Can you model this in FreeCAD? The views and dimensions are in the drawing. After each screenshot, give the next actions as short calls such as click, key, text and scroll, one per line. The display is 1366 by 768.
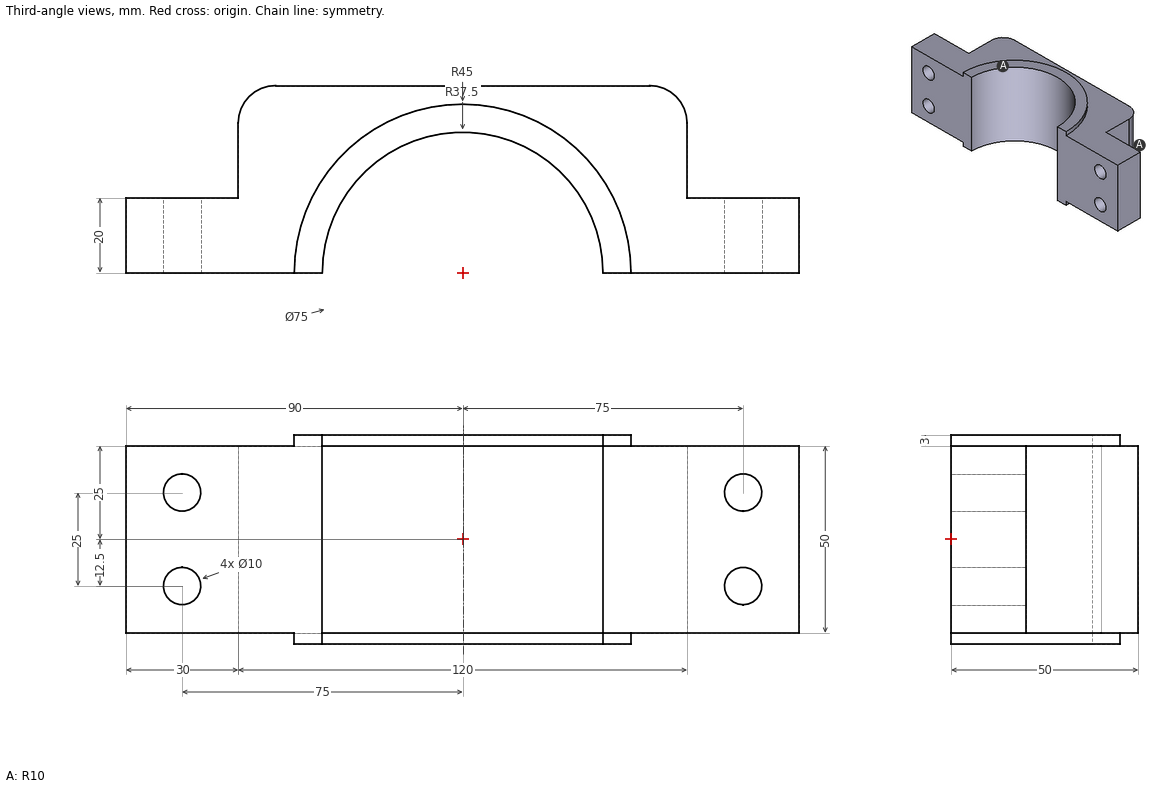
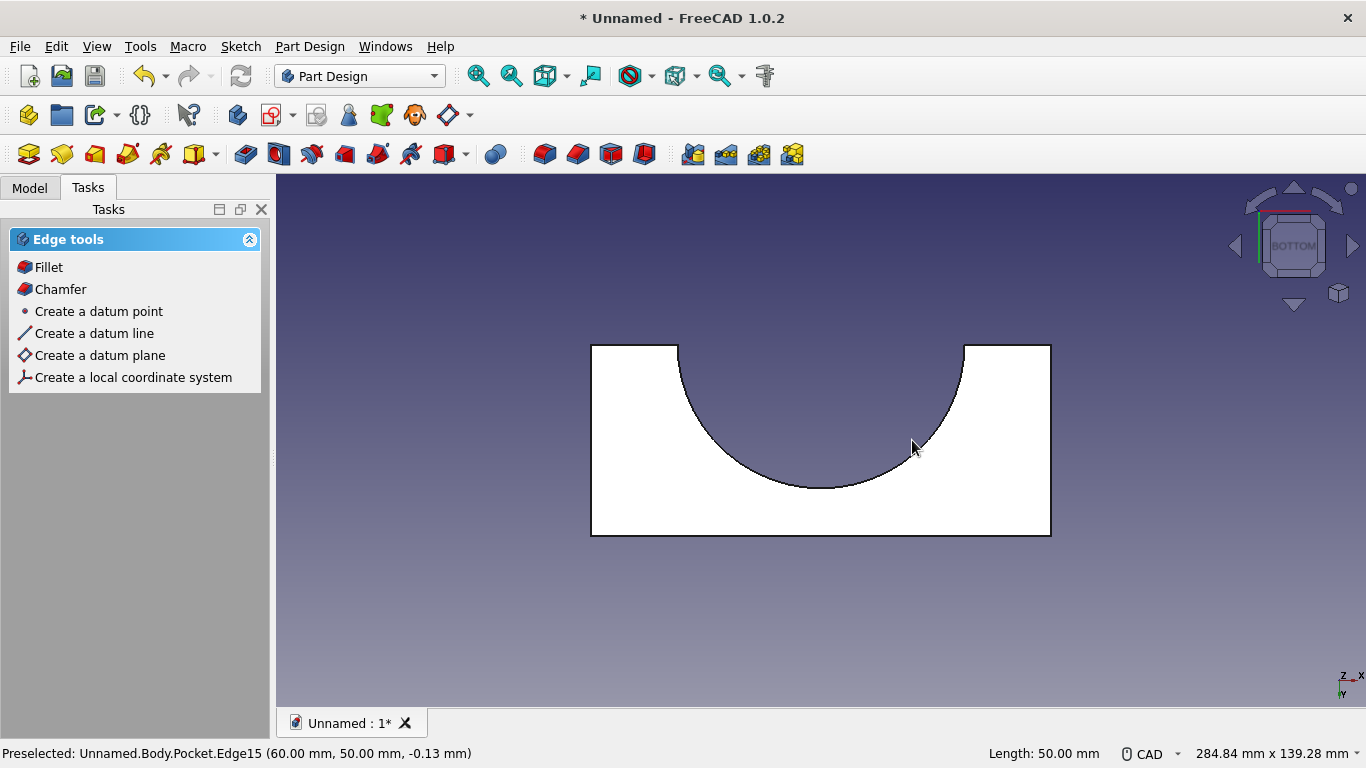
key(v)
key(f)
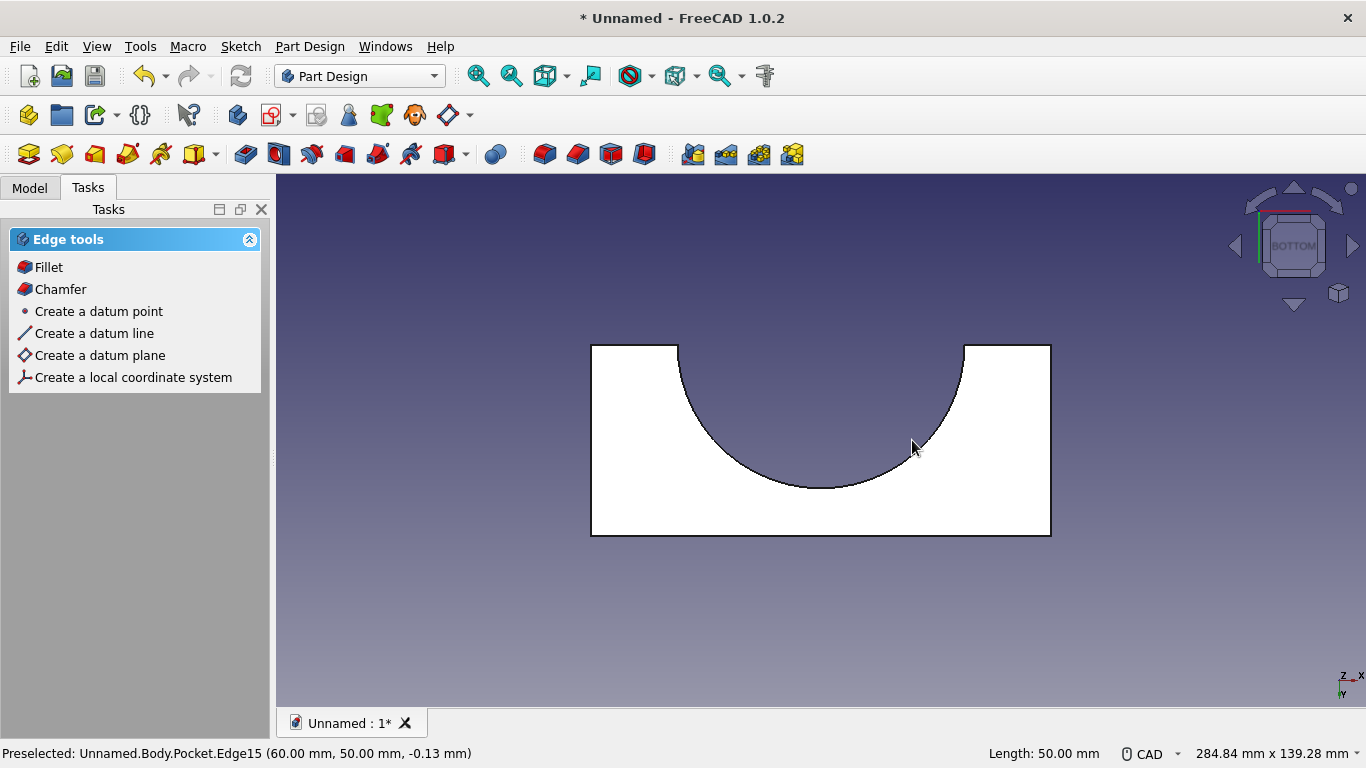
key(4)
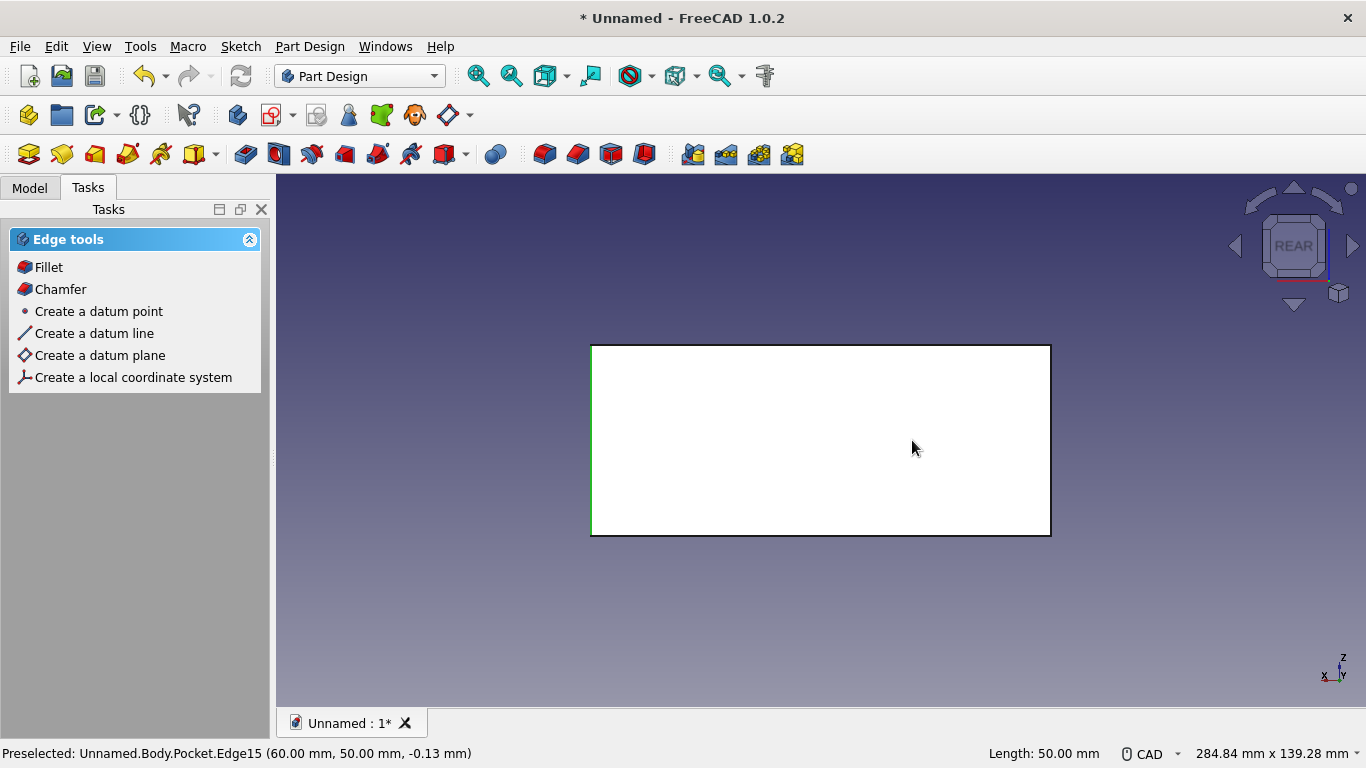
key(v)
key(f)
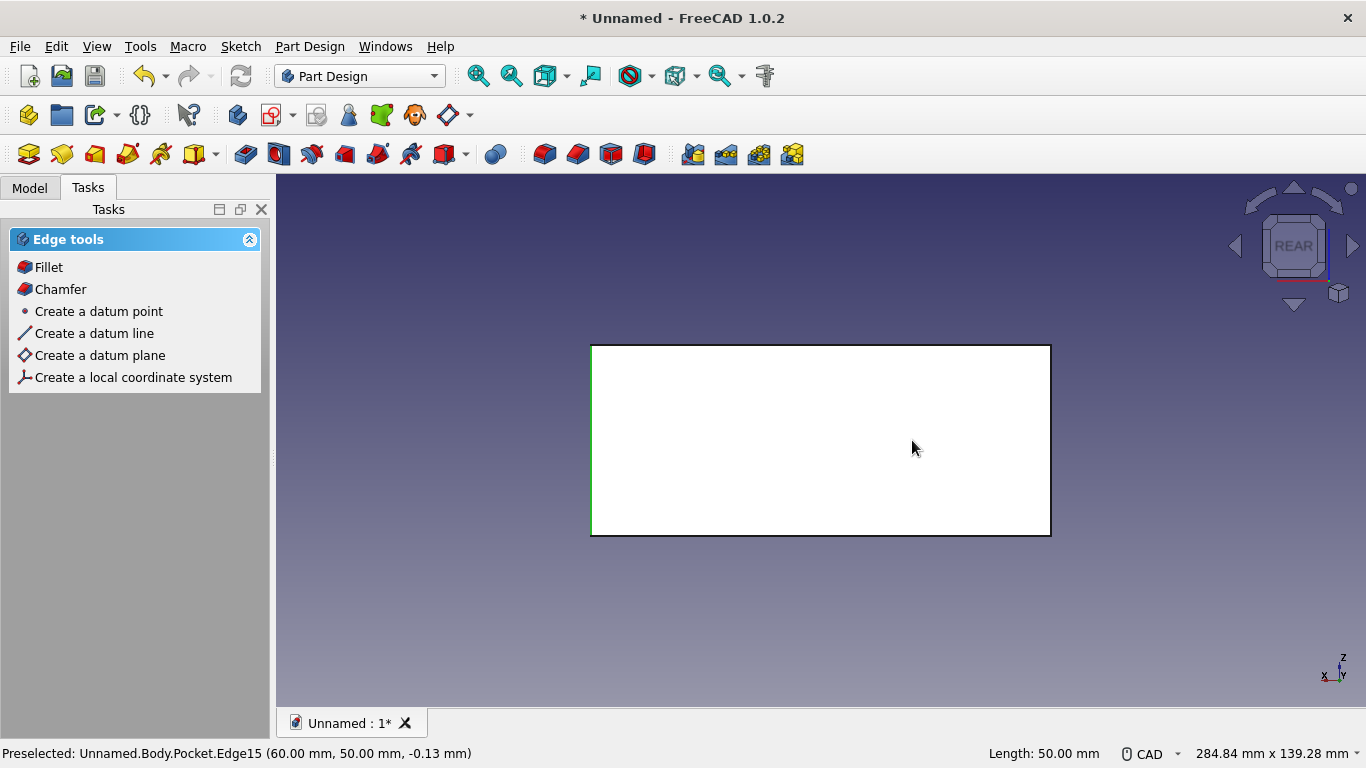
click(1051, 440, ctrl)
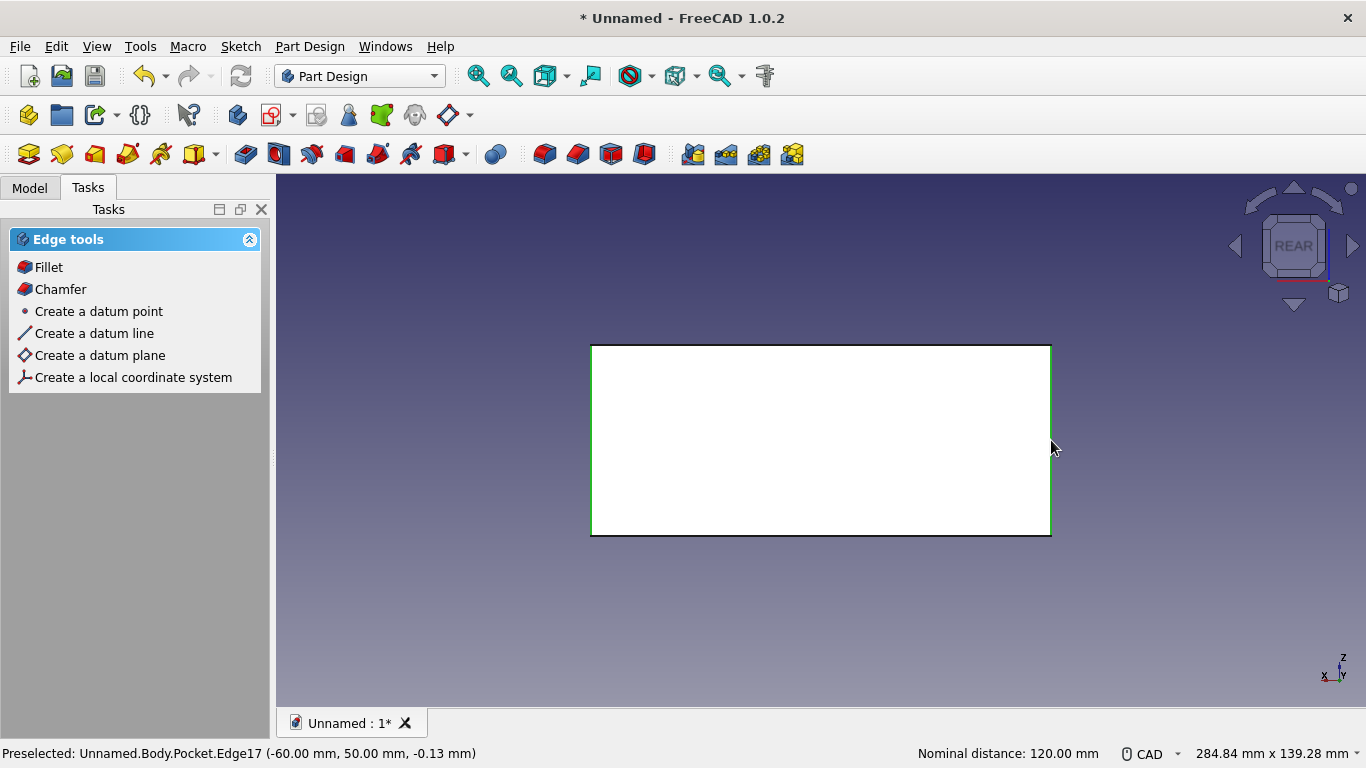
click(545, 154)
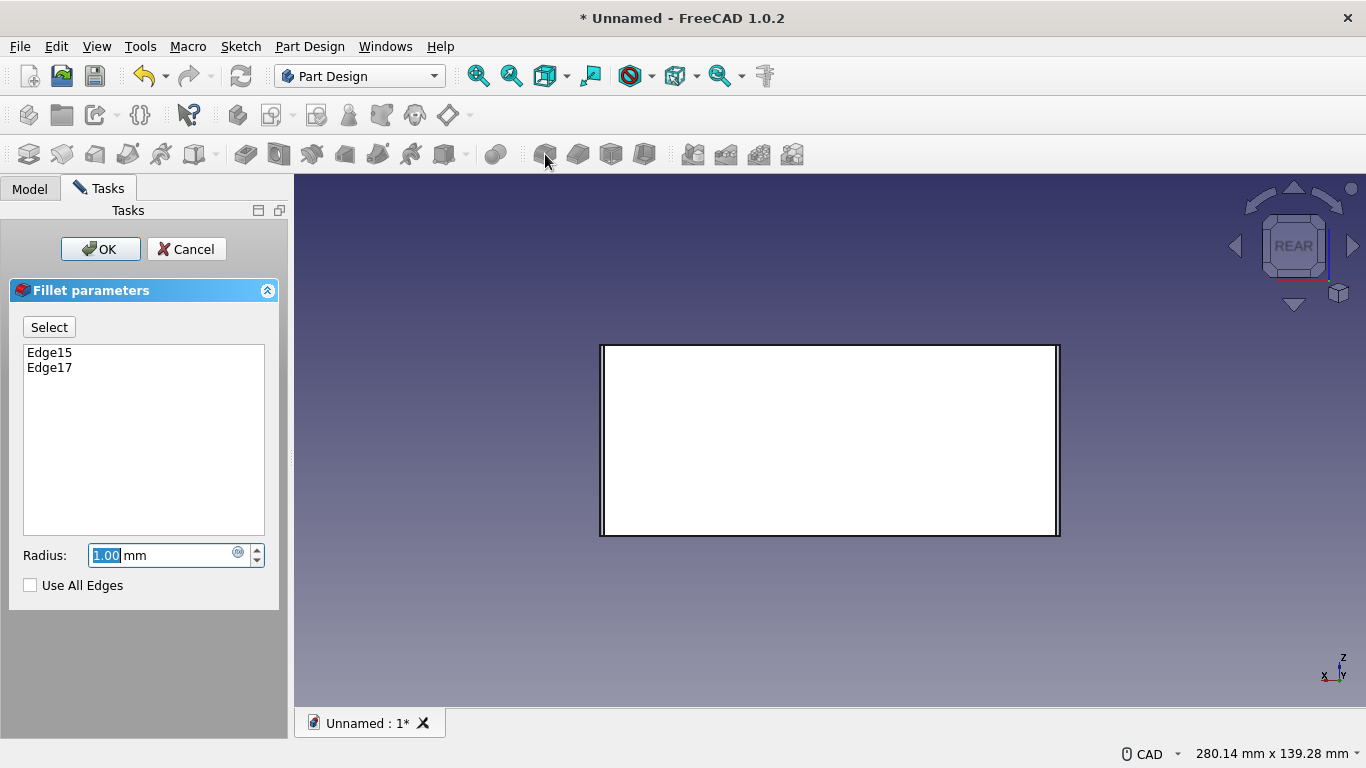
text(10)
key(Tab)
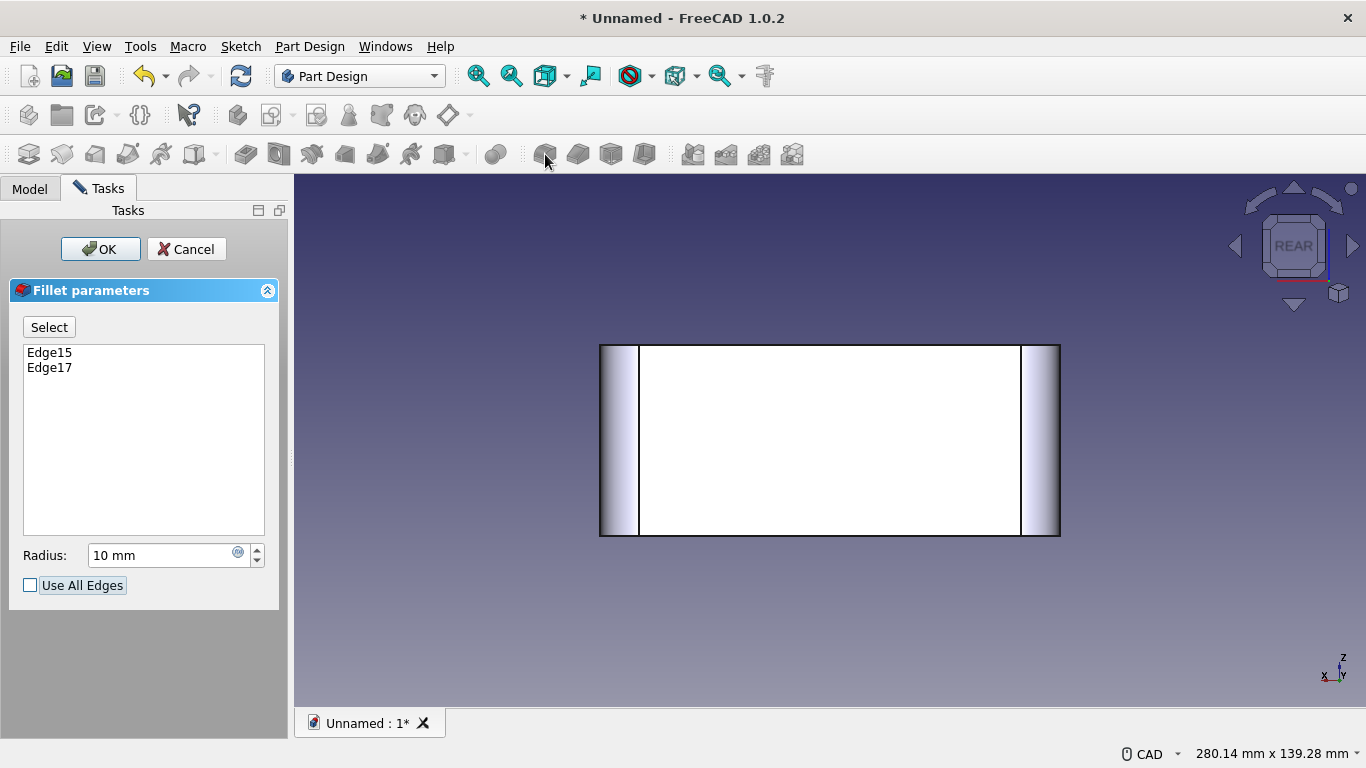
click(101, 249)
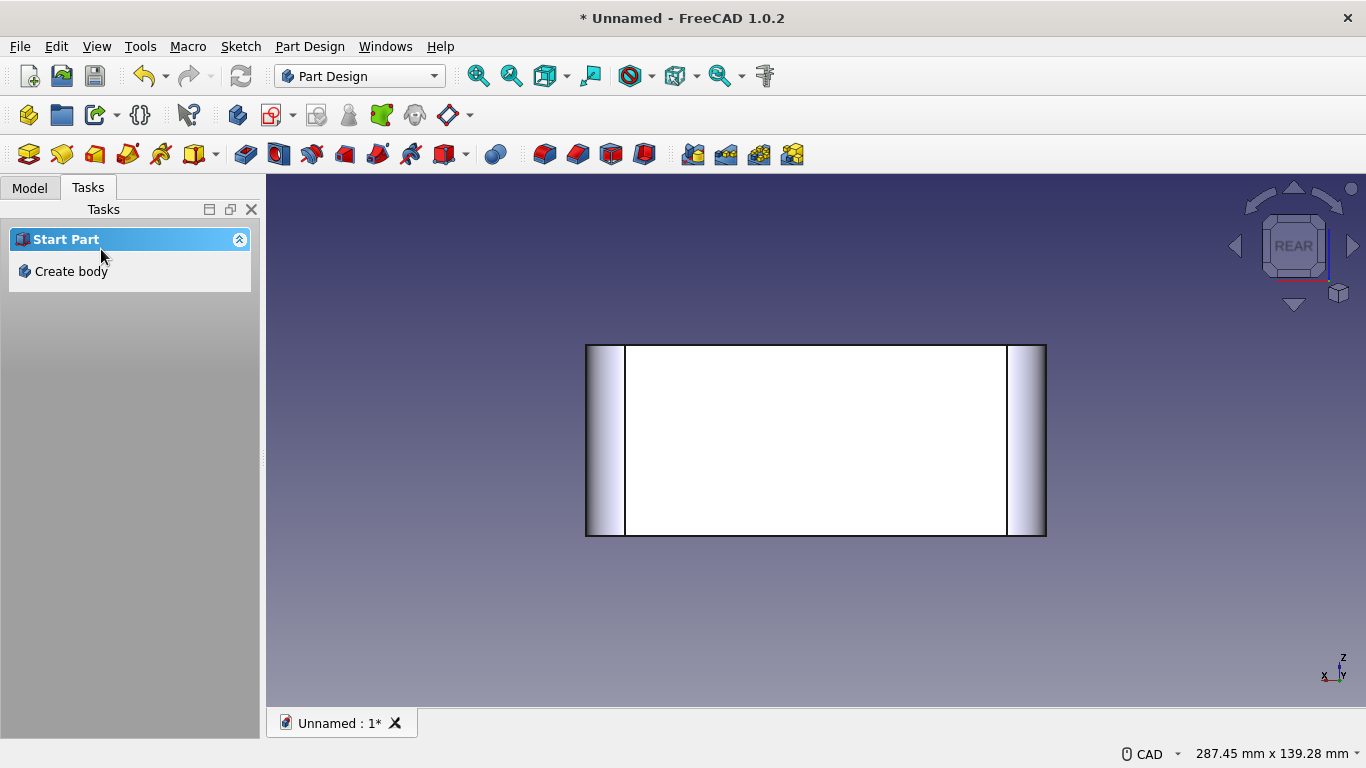
key(v)
key(f)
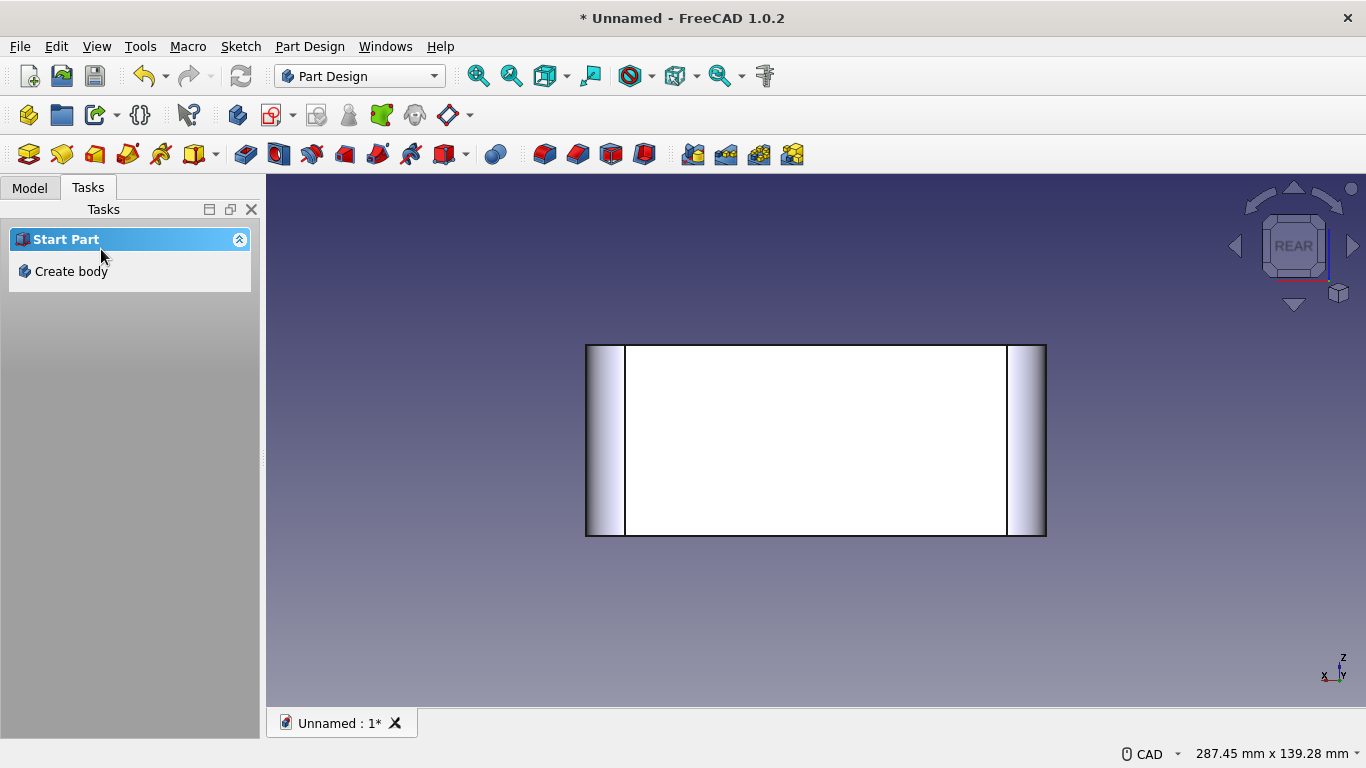
click(270, 116)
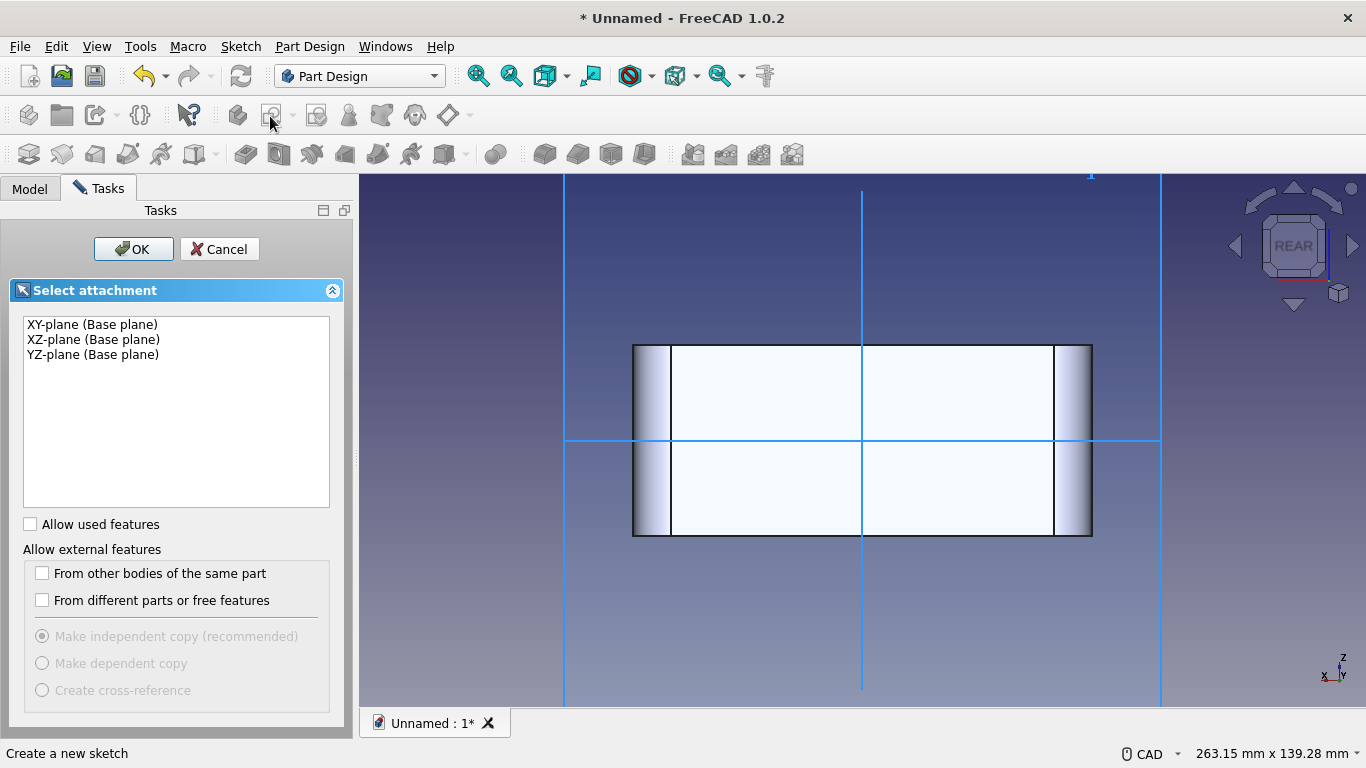
click(84, 340)